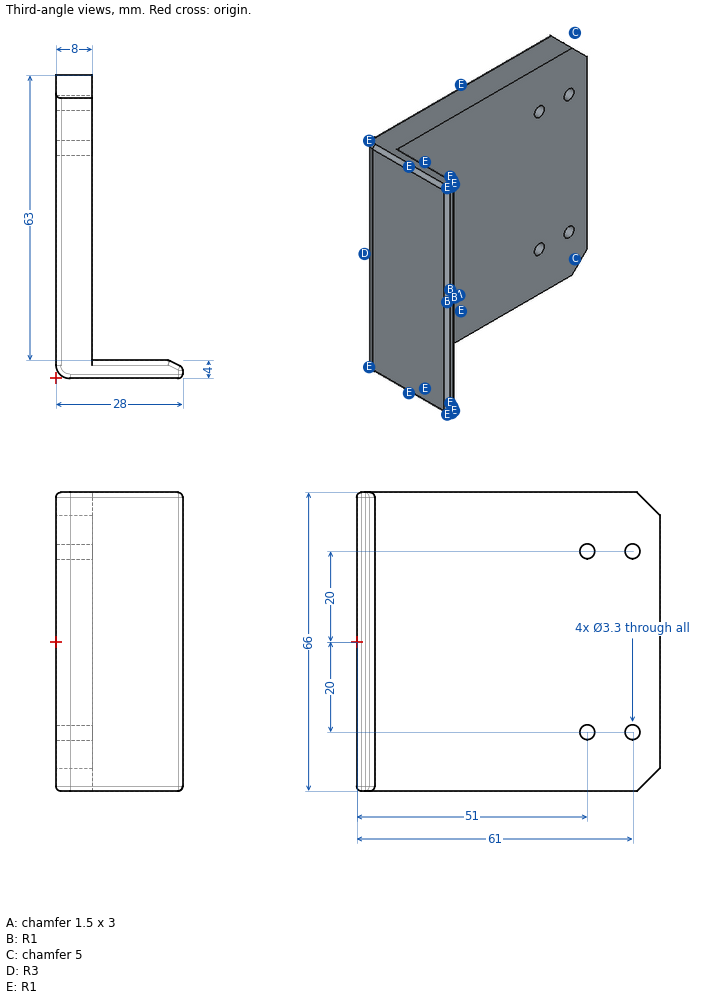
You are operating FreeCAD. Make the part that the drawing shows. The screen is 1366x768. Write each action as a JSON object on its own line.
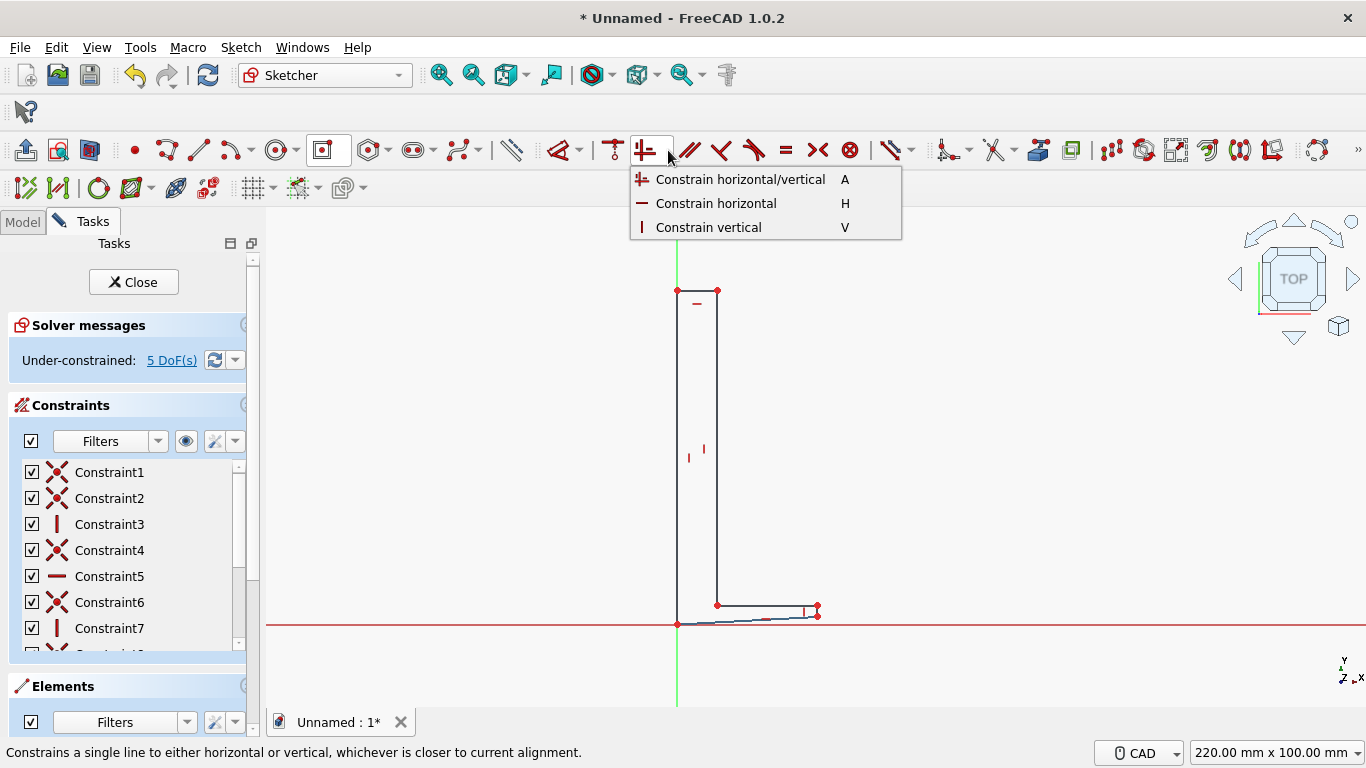
{"action": "left_click", "coordinate": [766, 203]}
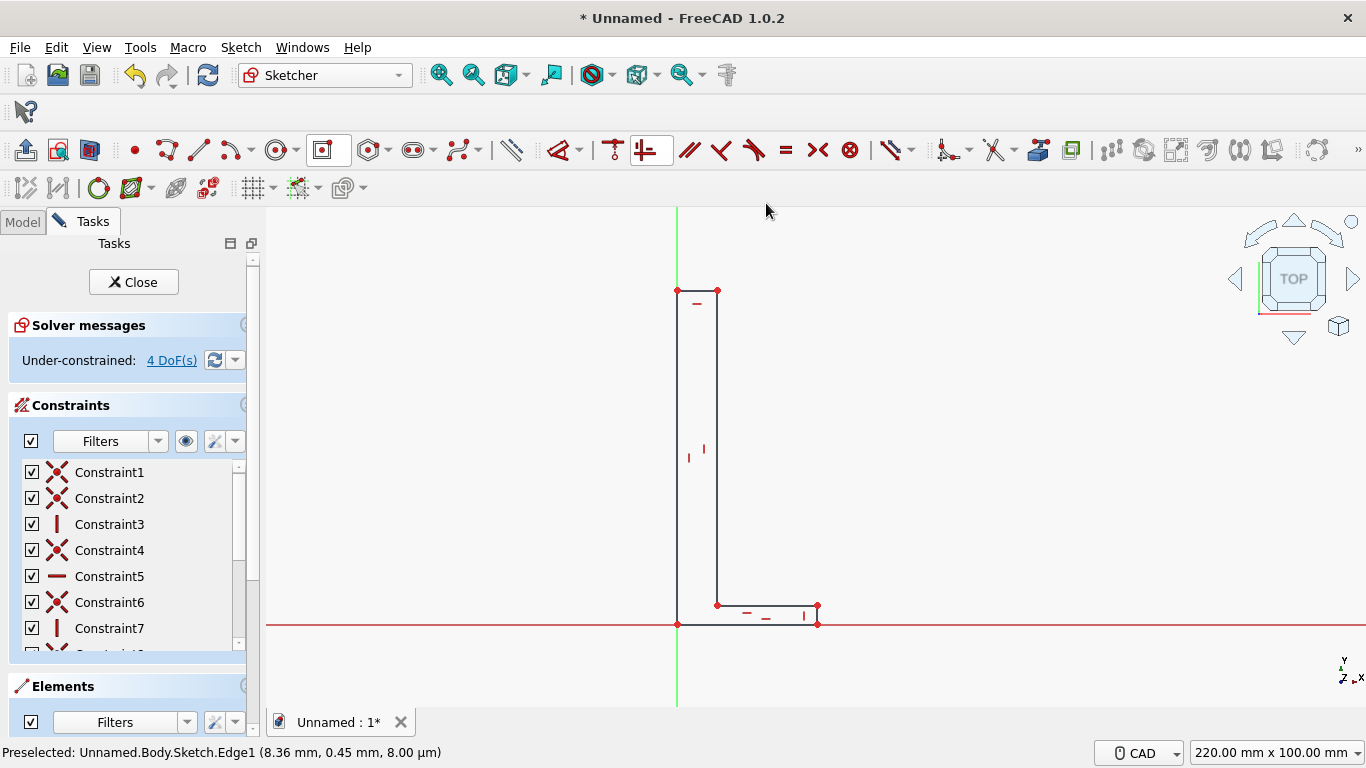
{"action": "left_click", "coordinate": [558, 150]}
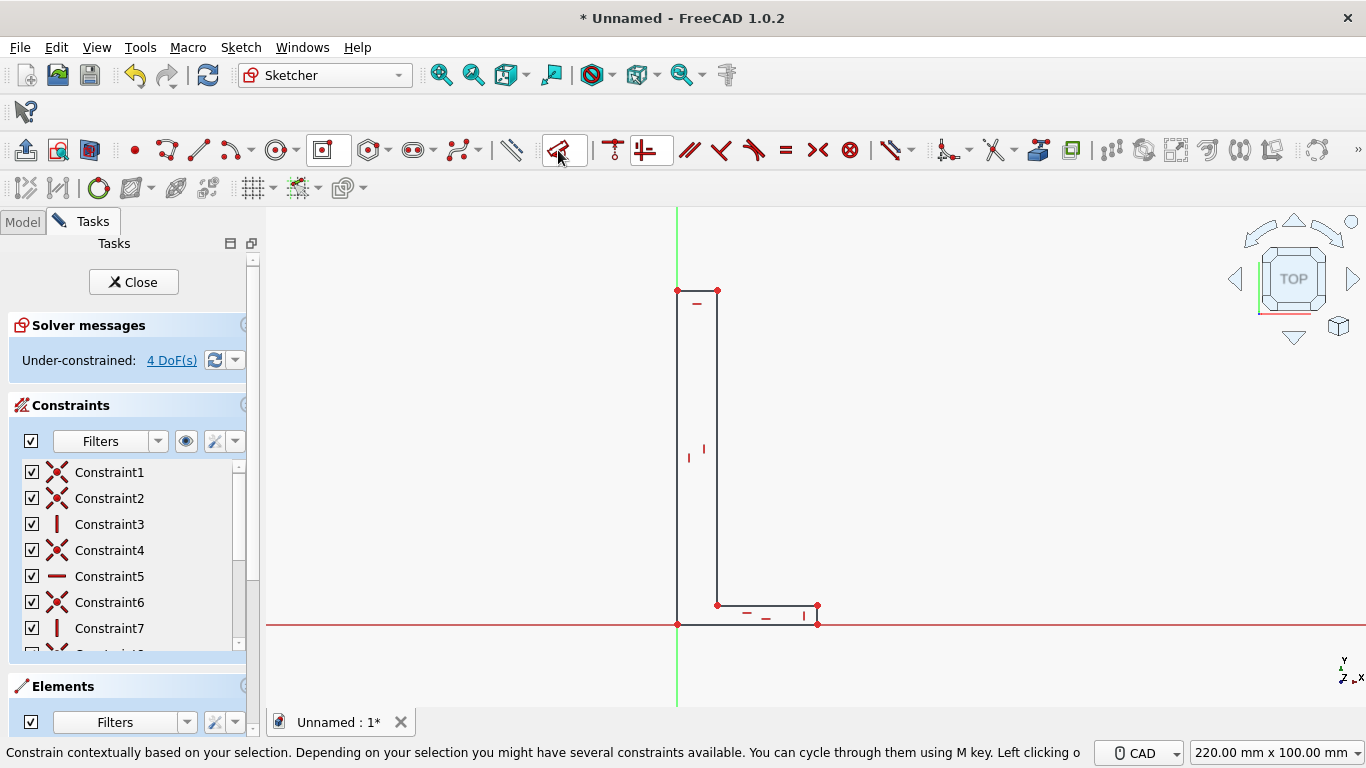
{"action": "scroll", "coordinate": [817, 615], "scroll_direction": "up", "scroll_amount": 4}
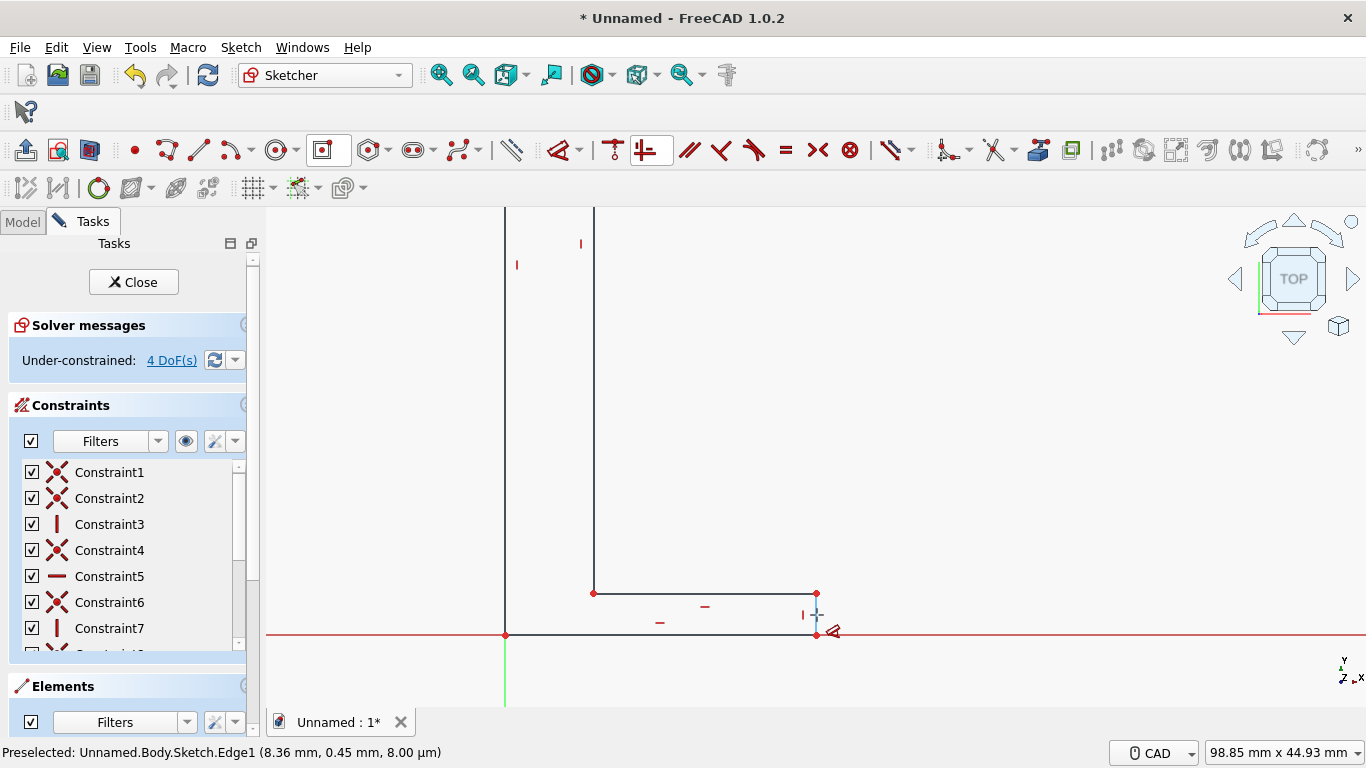
{"action": "left_click", "coordinate": [816, 615]}
{"action": "left_click", "coordinate": [850, 615]}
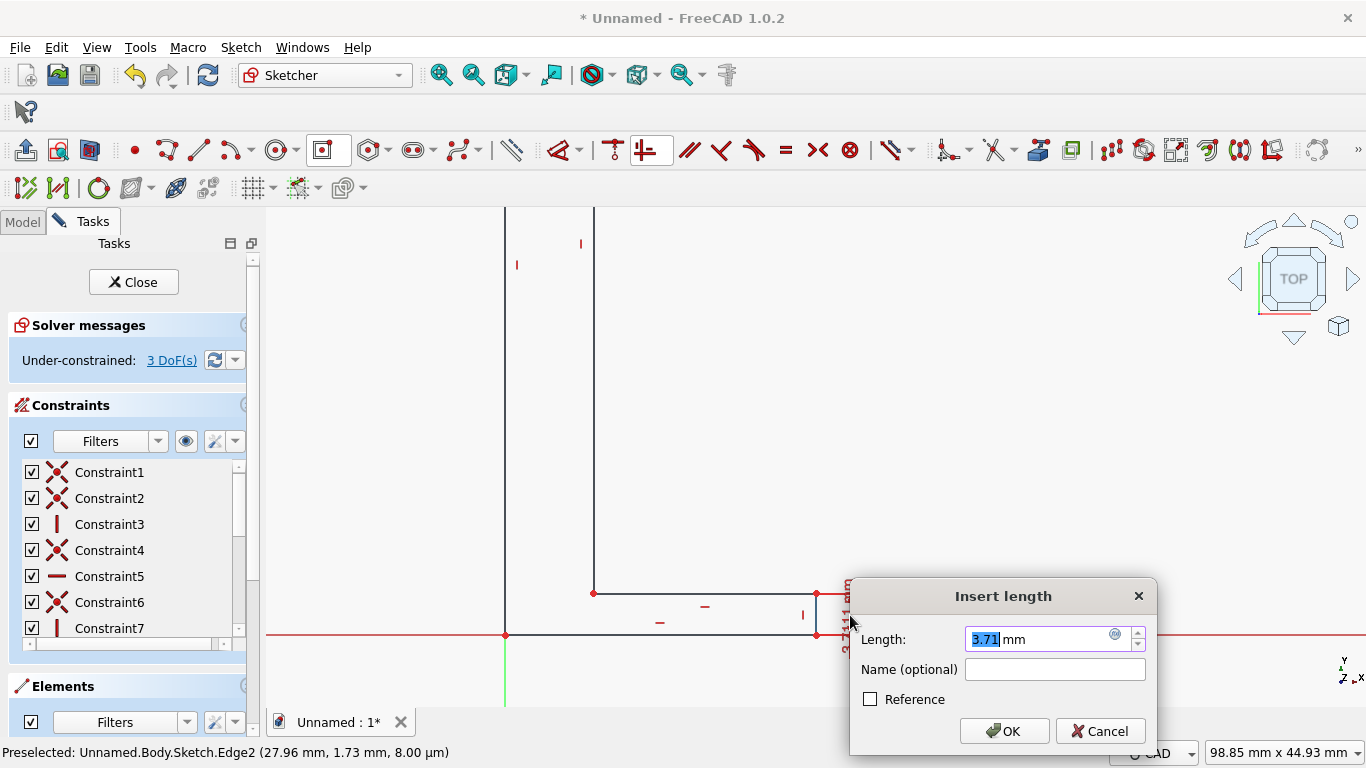
{"action": "type", "text": "4"}
{"action": "key", "text": "Return"}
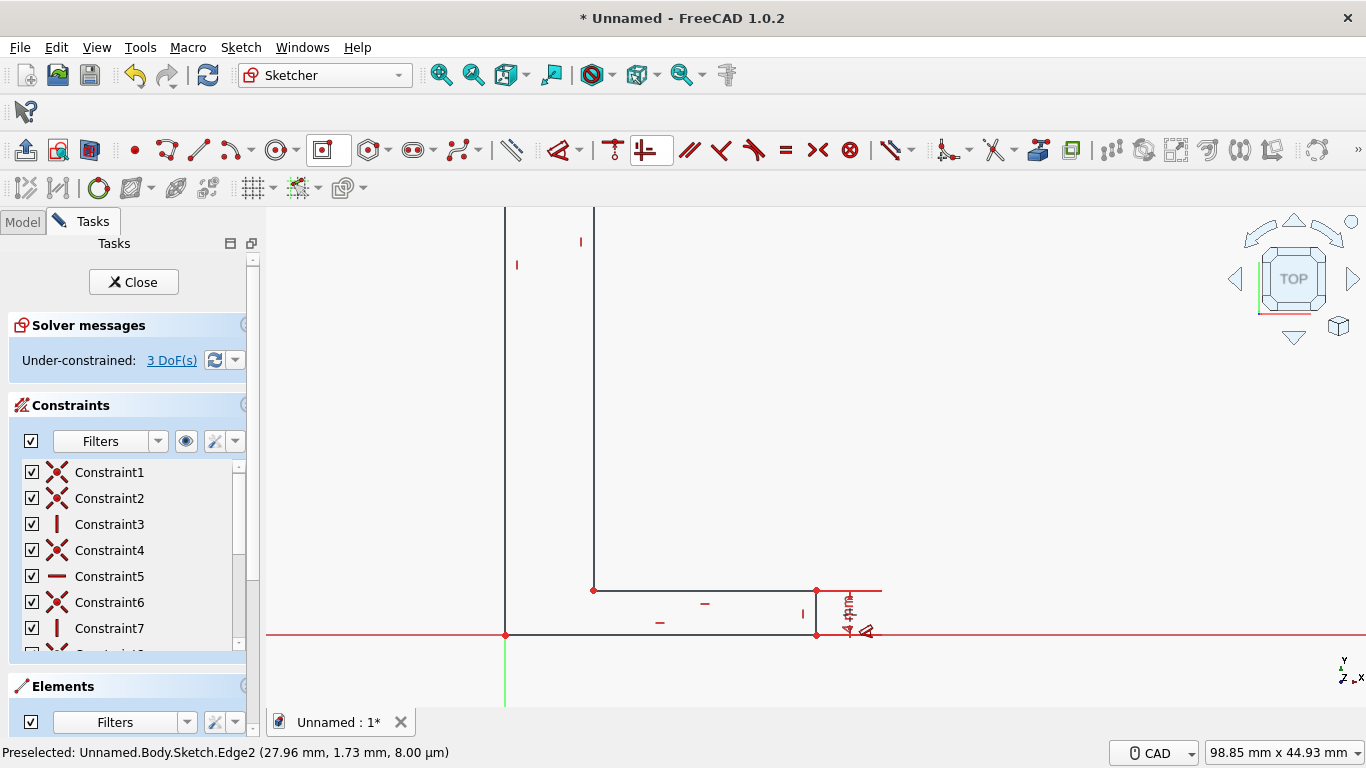
{"action": "scroll", "coordinate": [818, 616], "scroll_direction": "down", "scroll_amount": 4}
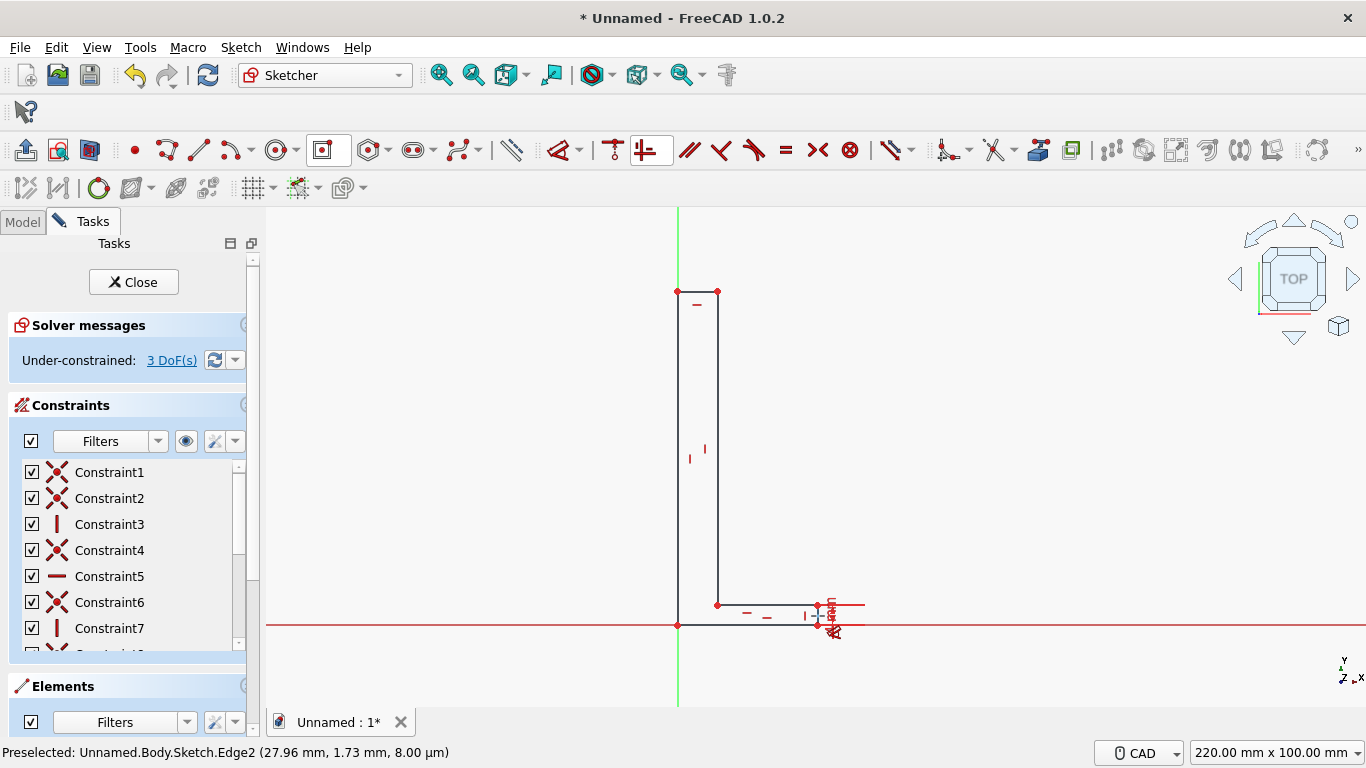
{"action": "left_click", "coordinate": [706, 292]}
{"action": "left_click", "coordinate": [698, 258]}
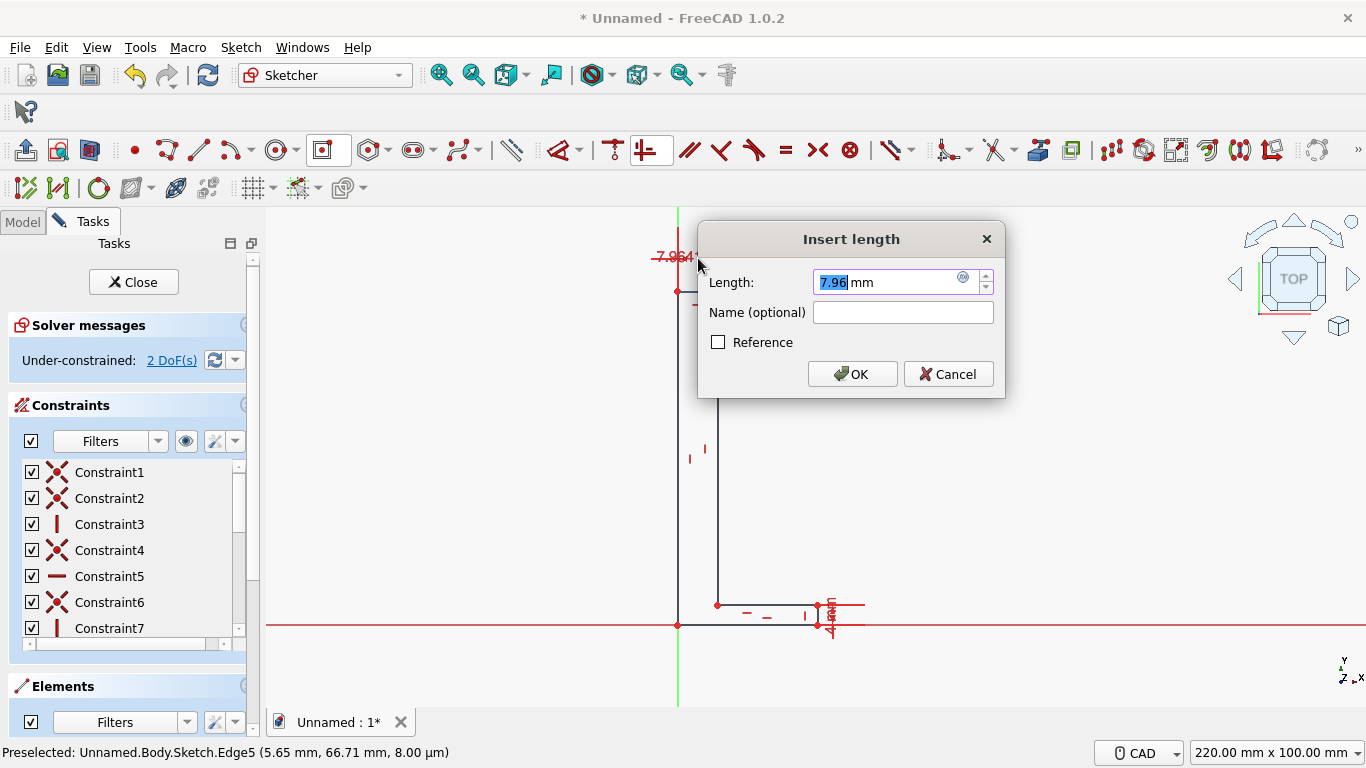
{"action": "type", "text": "8"}
{"action": "key", "text": "Return"}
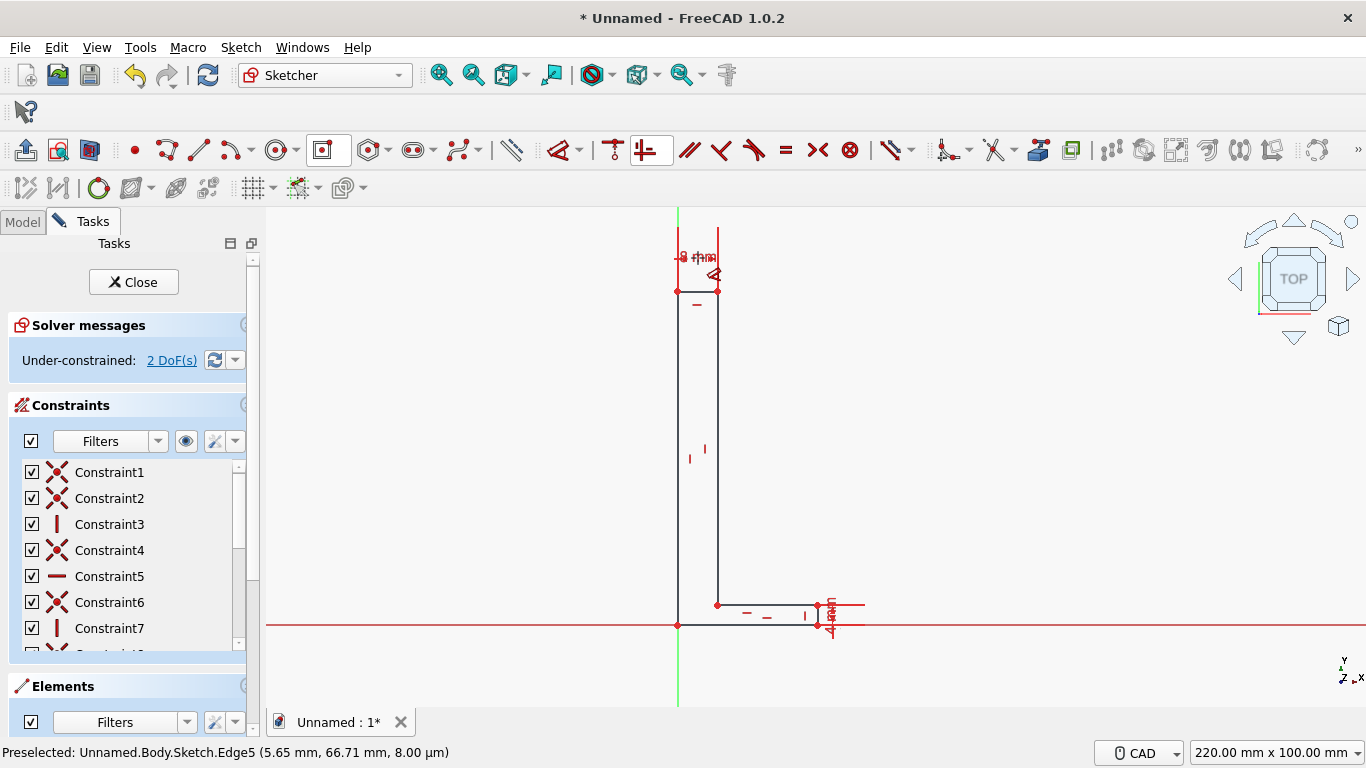
{"action": "left_click", "coordinate": [720, 625]}
{"action": "left_click", "coordinate": [748, 659]}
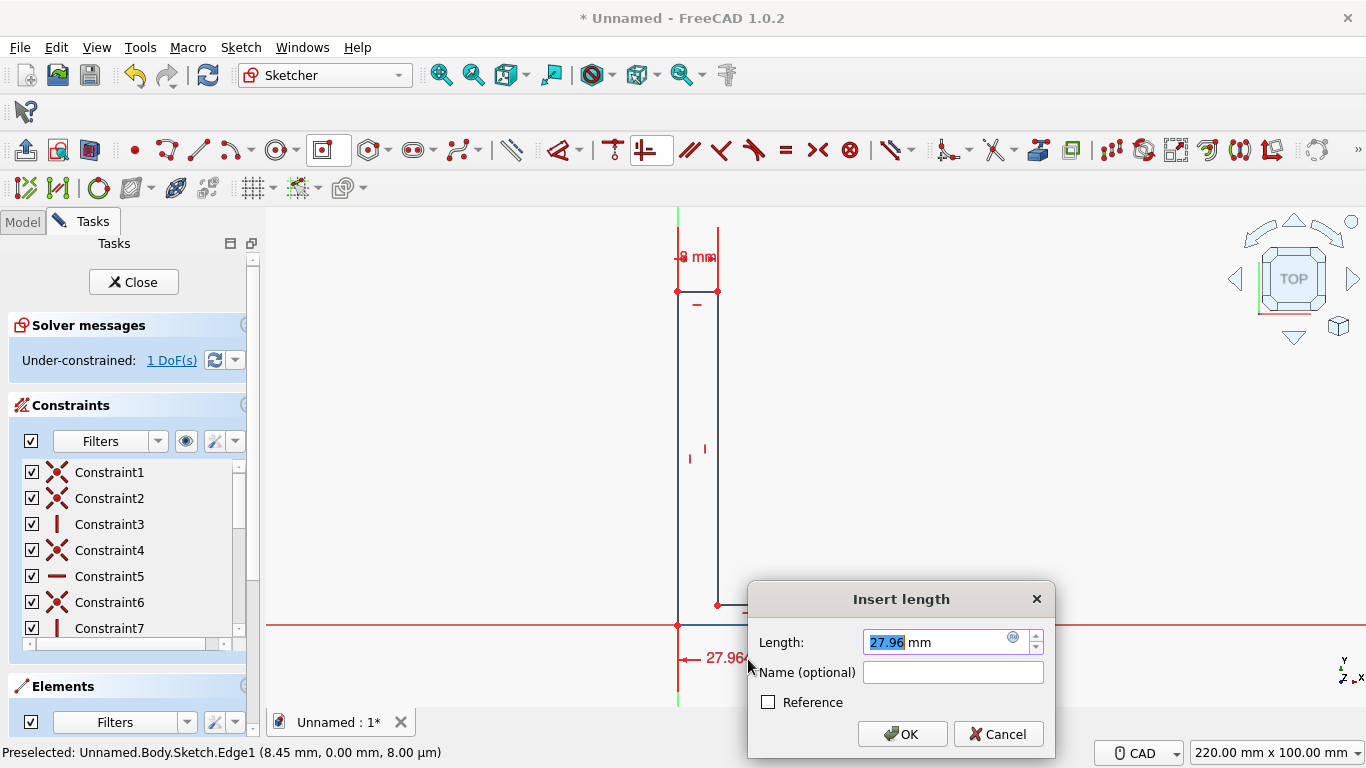
{"action": "type", "text": "28"}
{"action": "key", "text": "Return"}